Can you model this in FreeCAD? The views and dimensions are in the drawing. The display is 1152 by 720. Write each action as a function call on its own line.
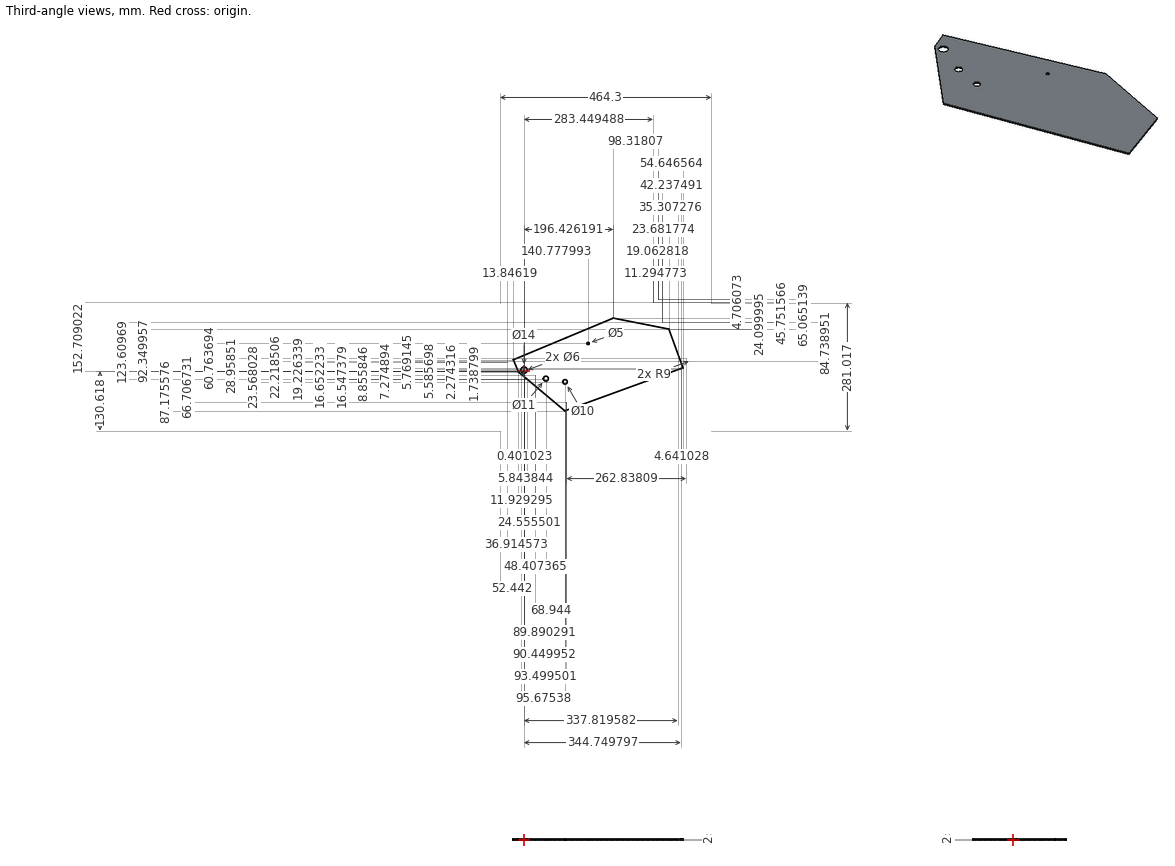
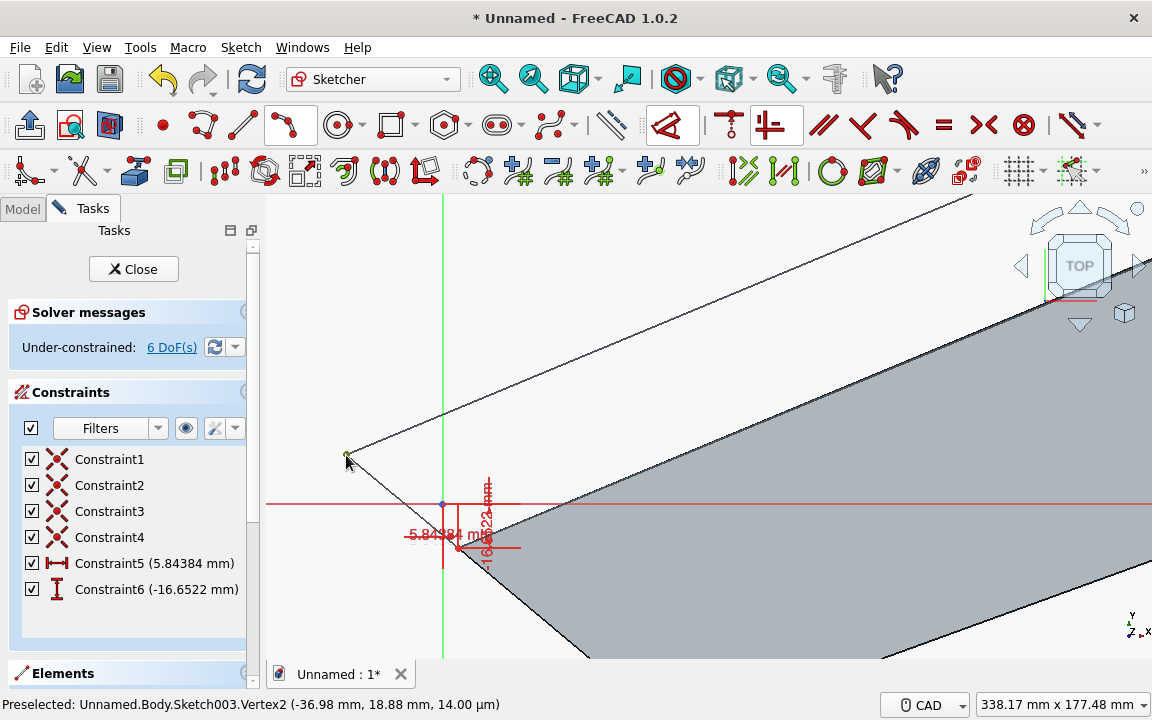
key(l)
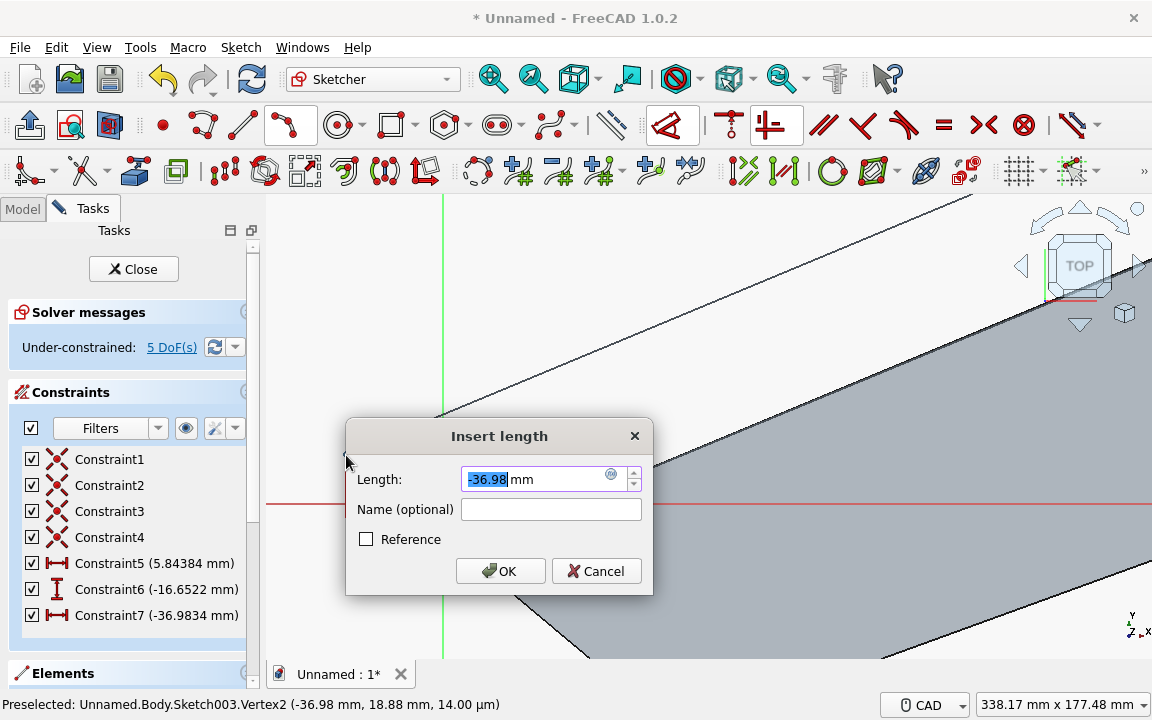
text(-36.914573)
key(Return)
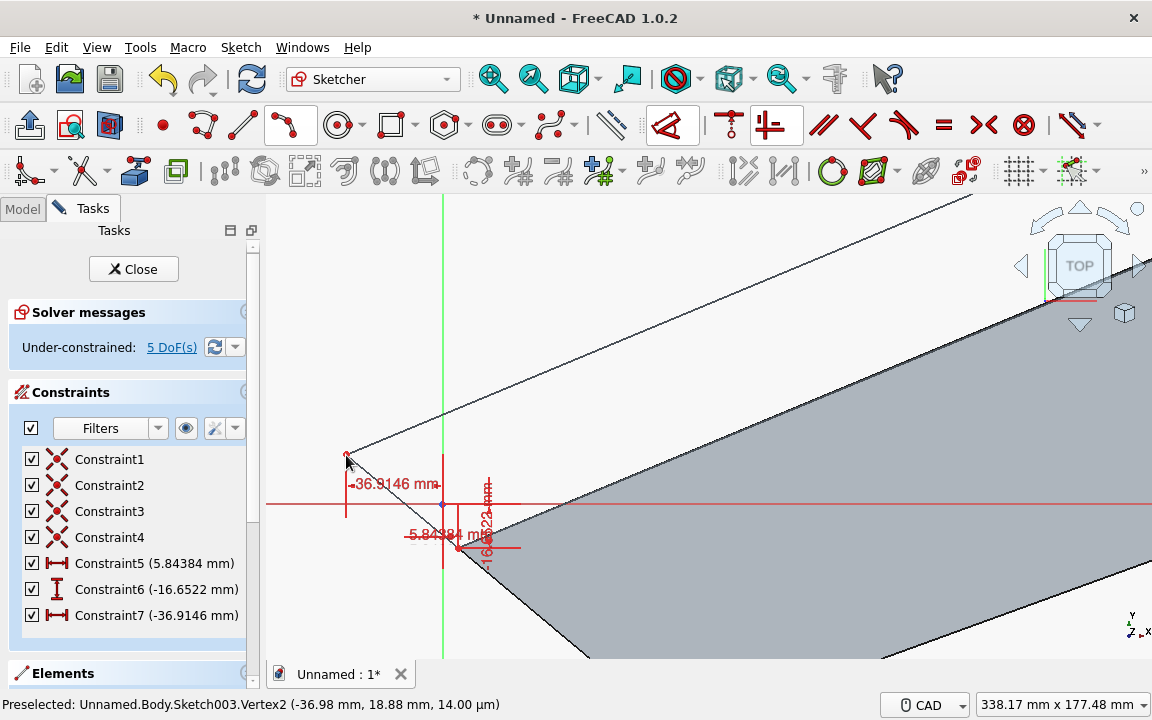
click(346, 455)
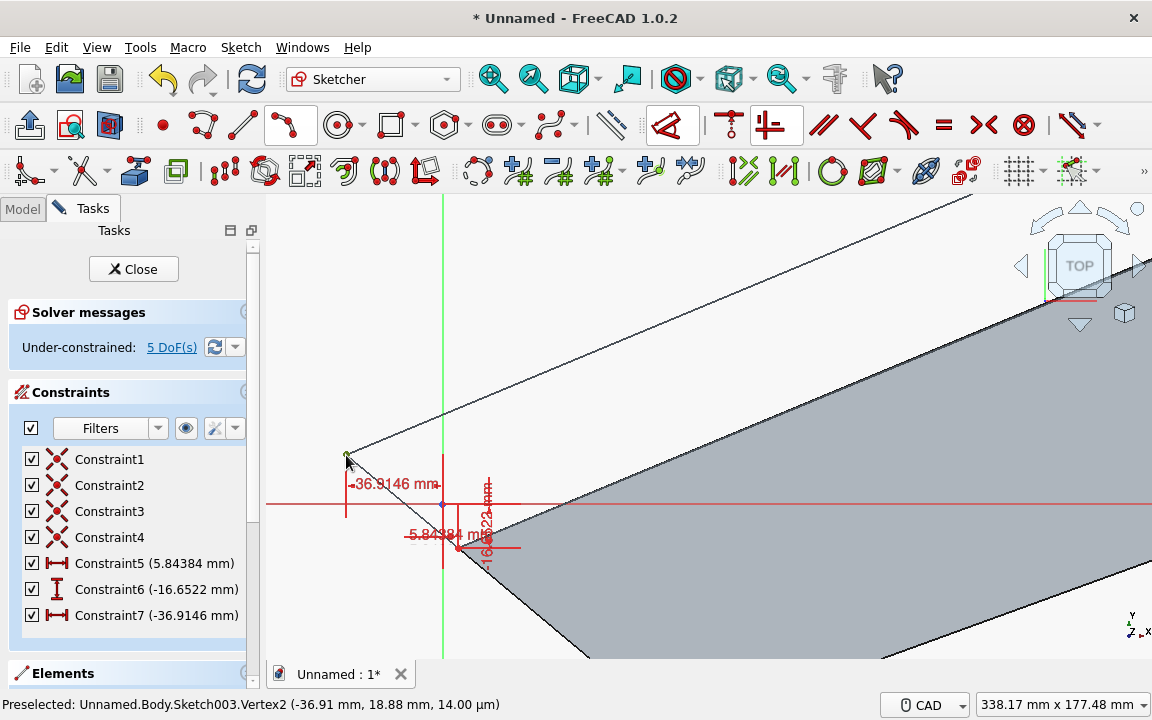
key(i)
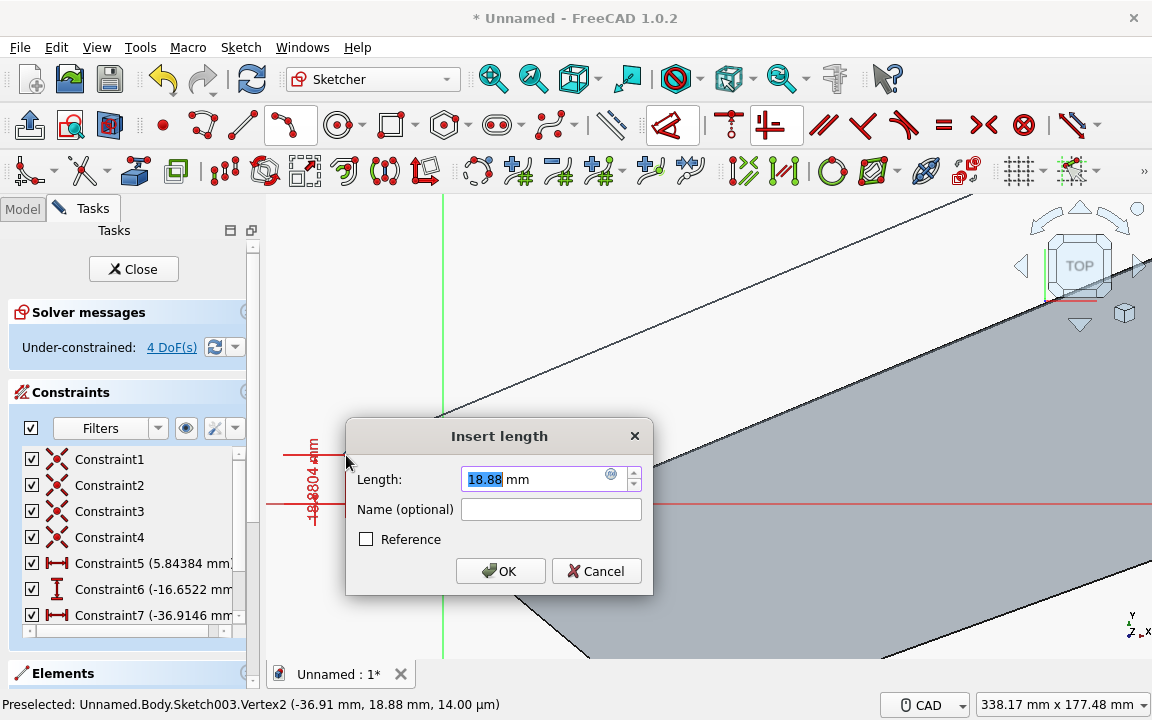
text(19.226339)
key(Return)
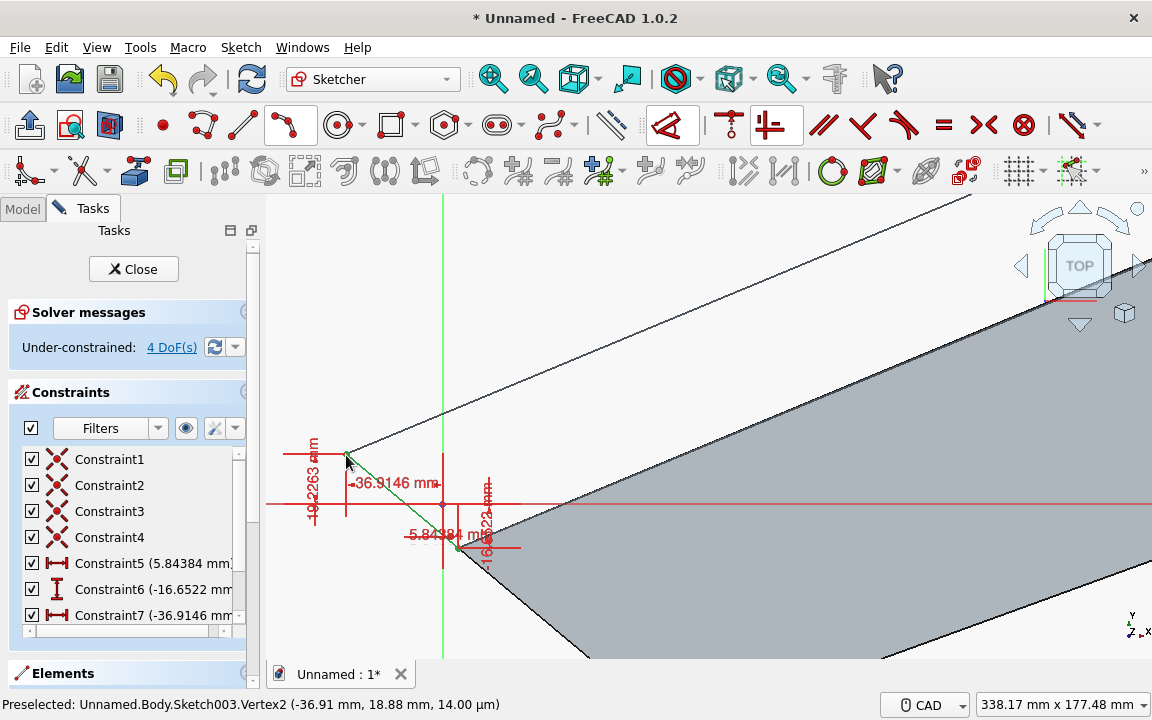
scroll(458, 548, down, 3)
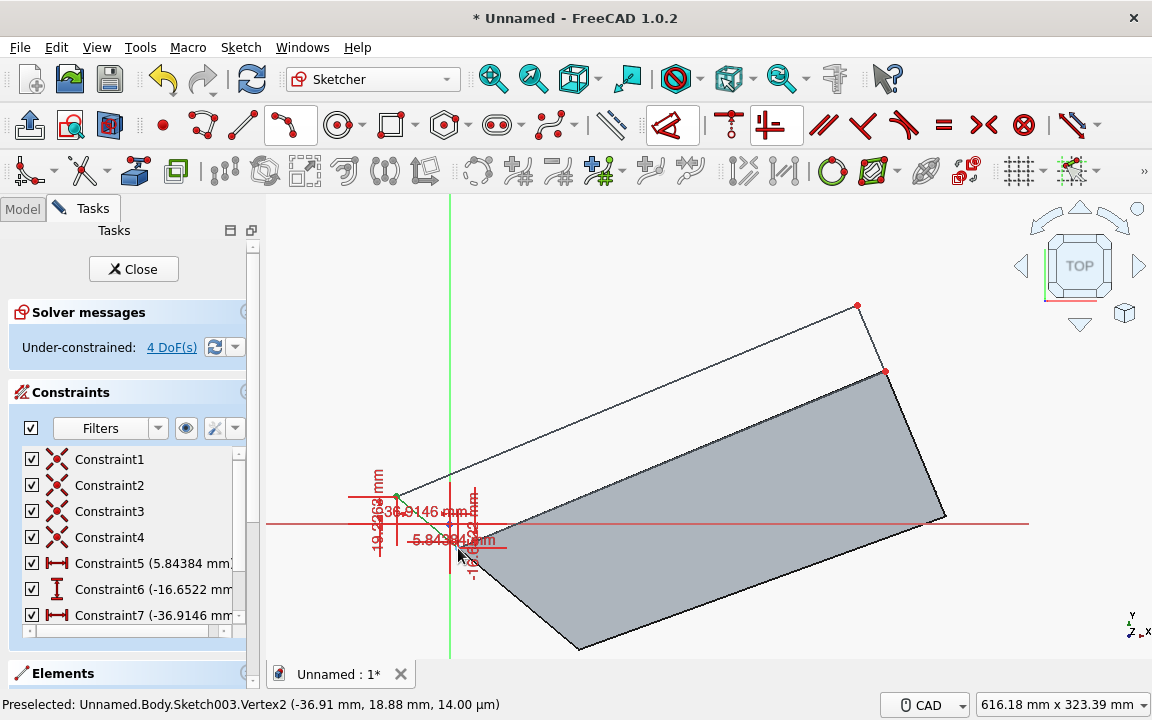
scroll(865, 325, up, 2)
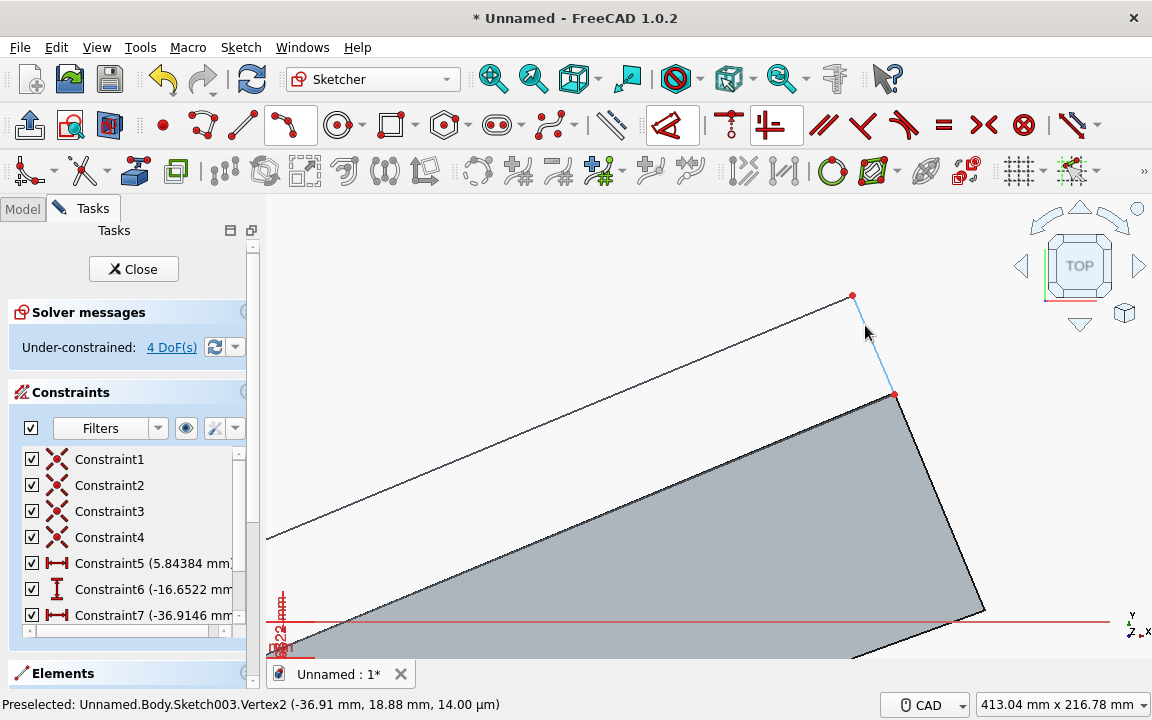
click(865, 325)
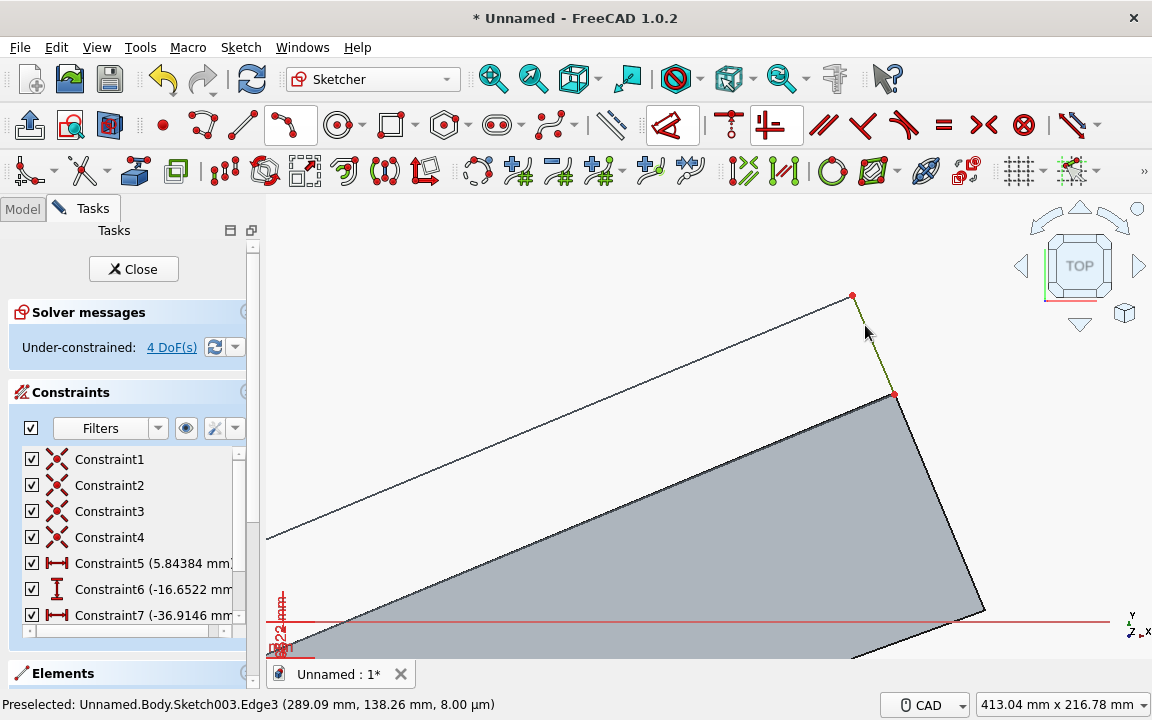
key(l)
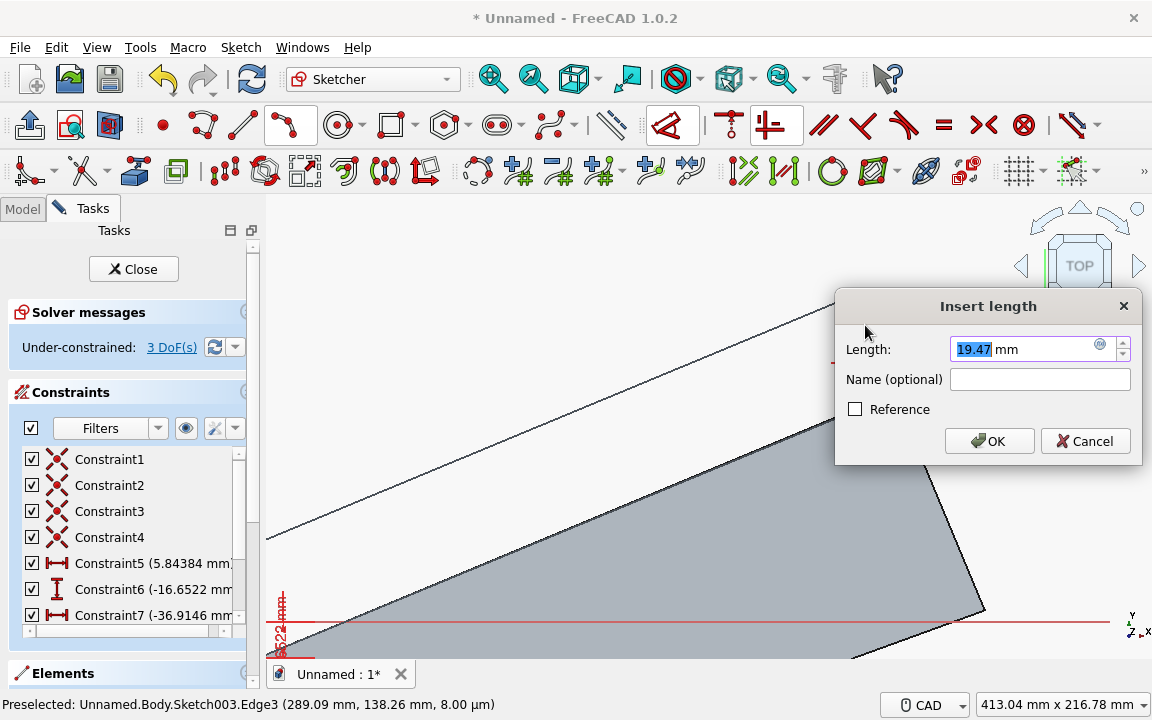
text(19.062818)
key(Return)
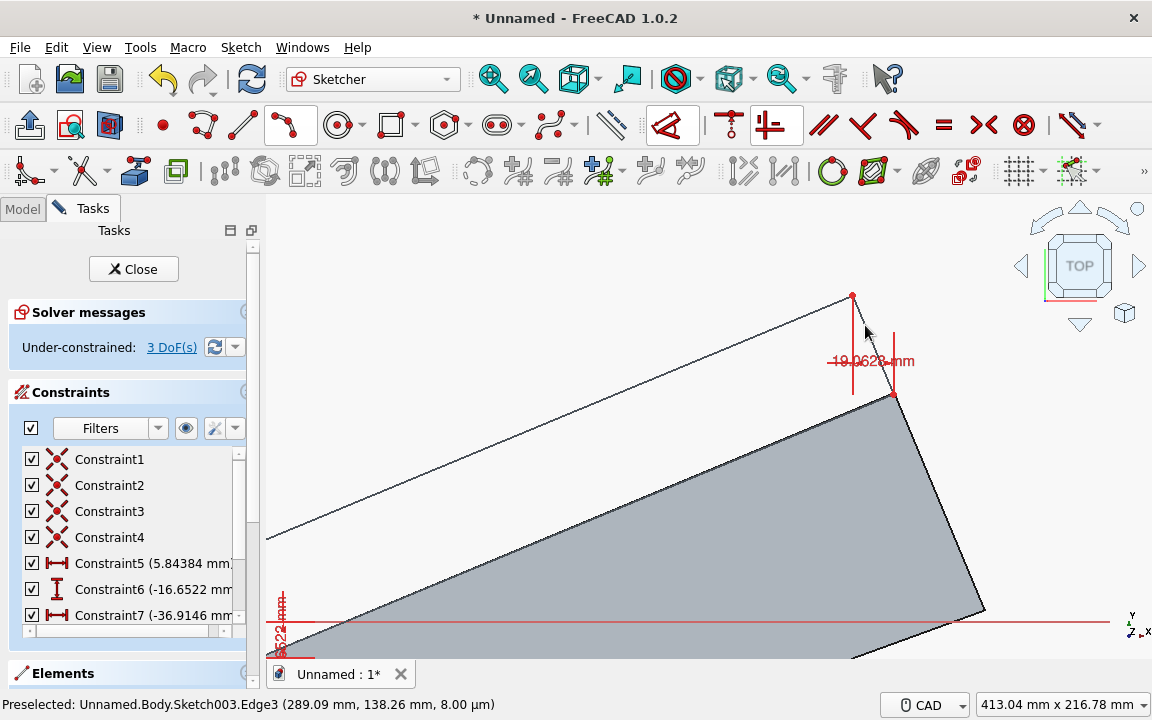
click(865, 325)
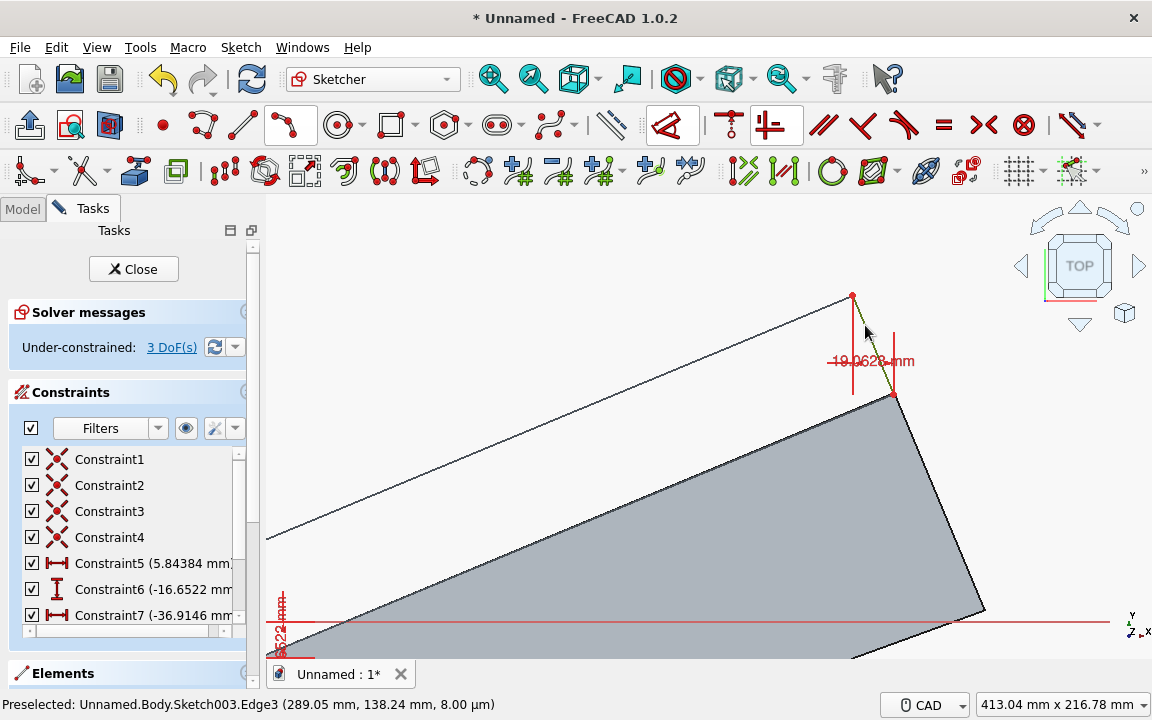
key(i)